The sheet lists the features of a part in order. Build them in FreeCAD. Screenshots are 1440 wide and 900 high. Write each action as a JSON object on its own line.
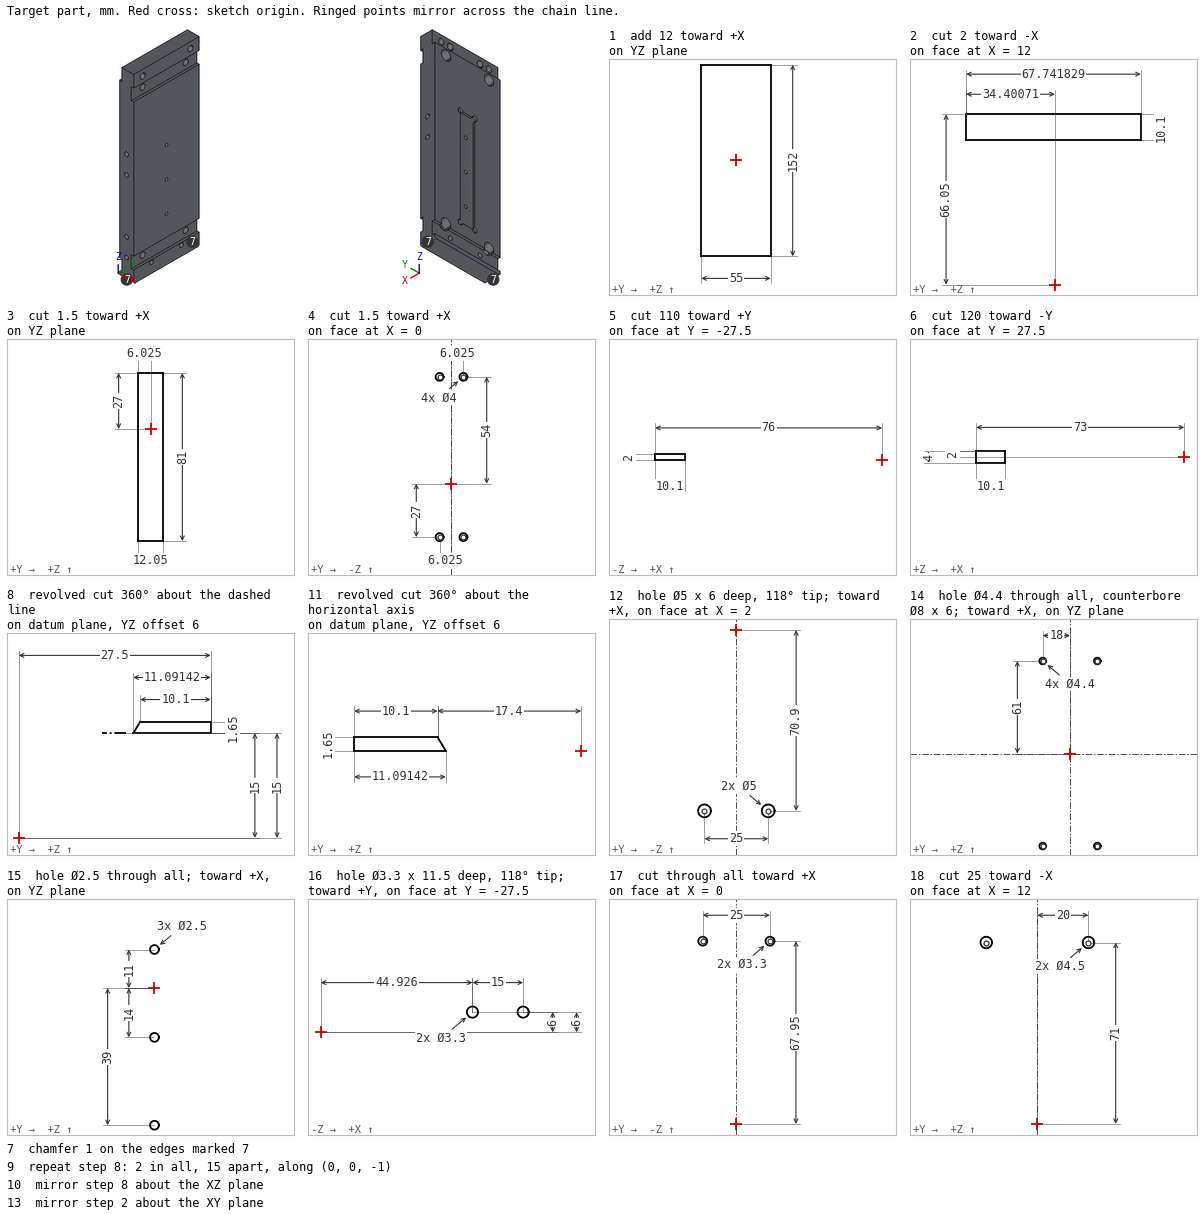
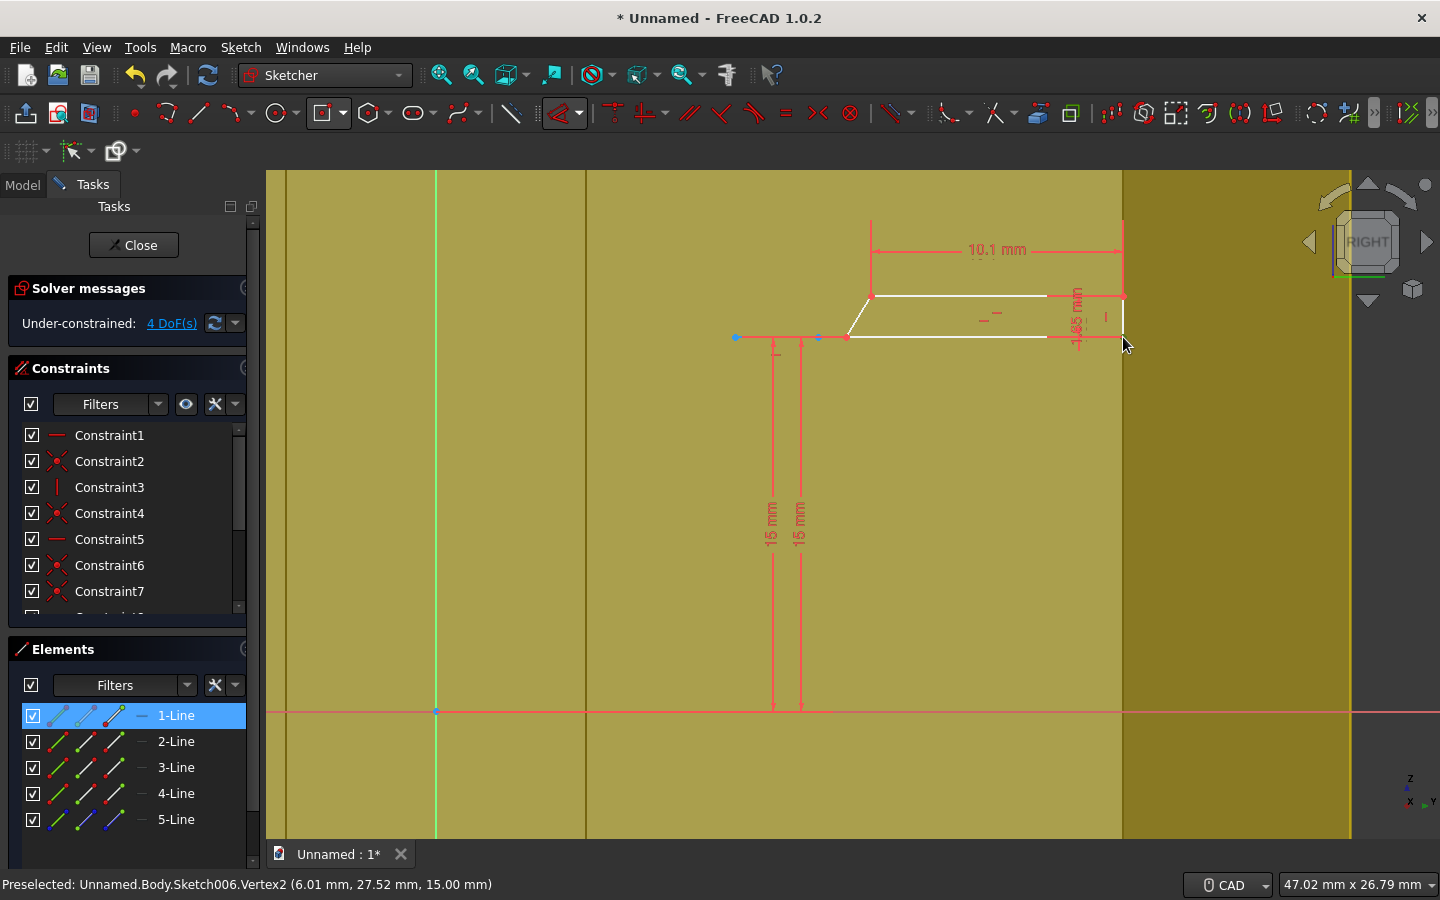
{"action": "left_click", "coordinate": [582, 114]}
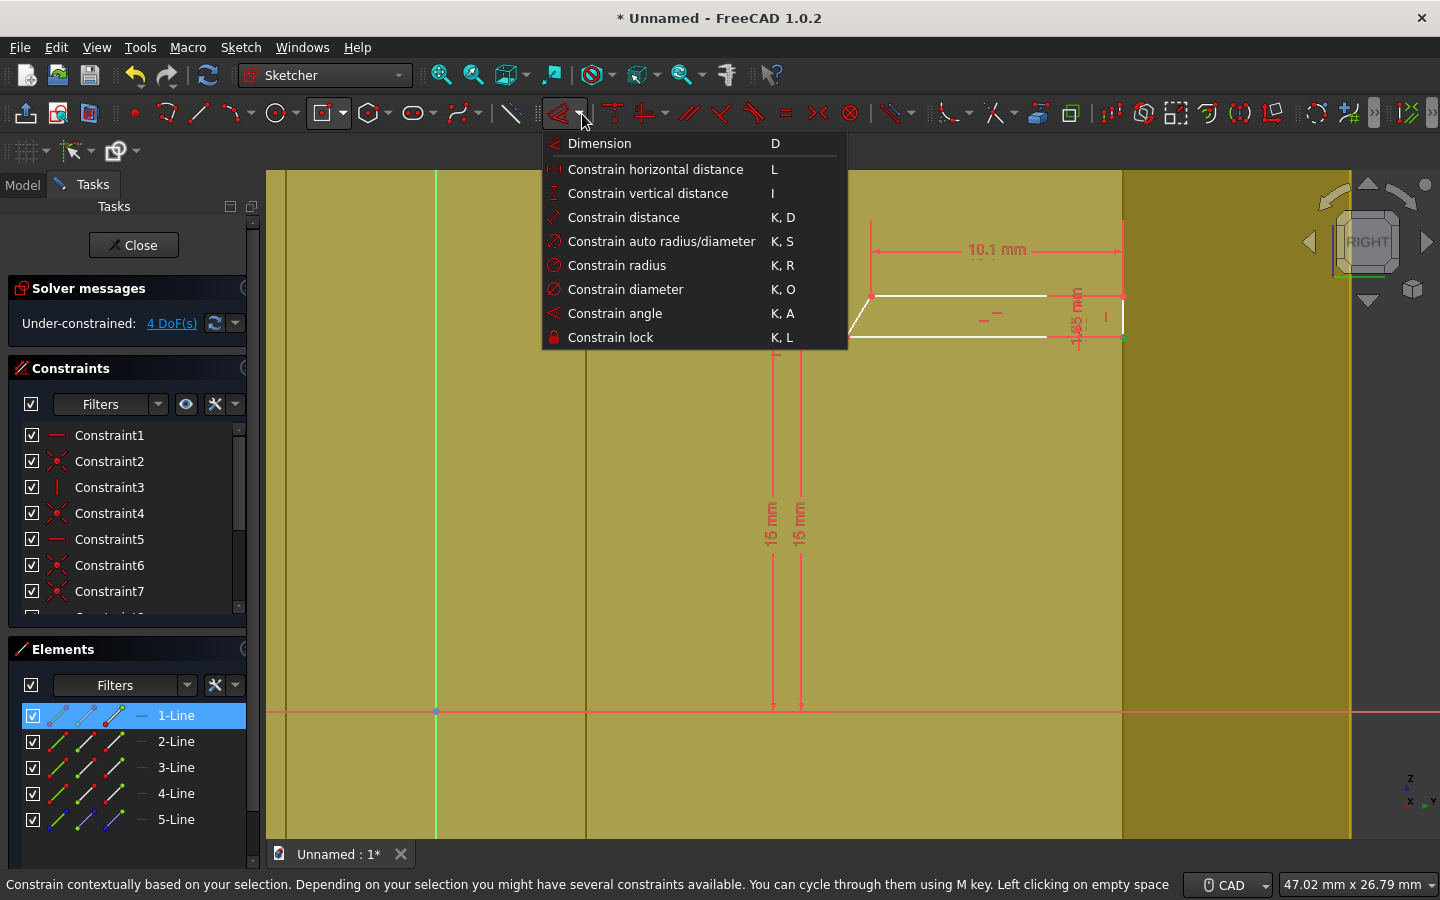
{"action": "left_click", "coordinate": [695, 169]}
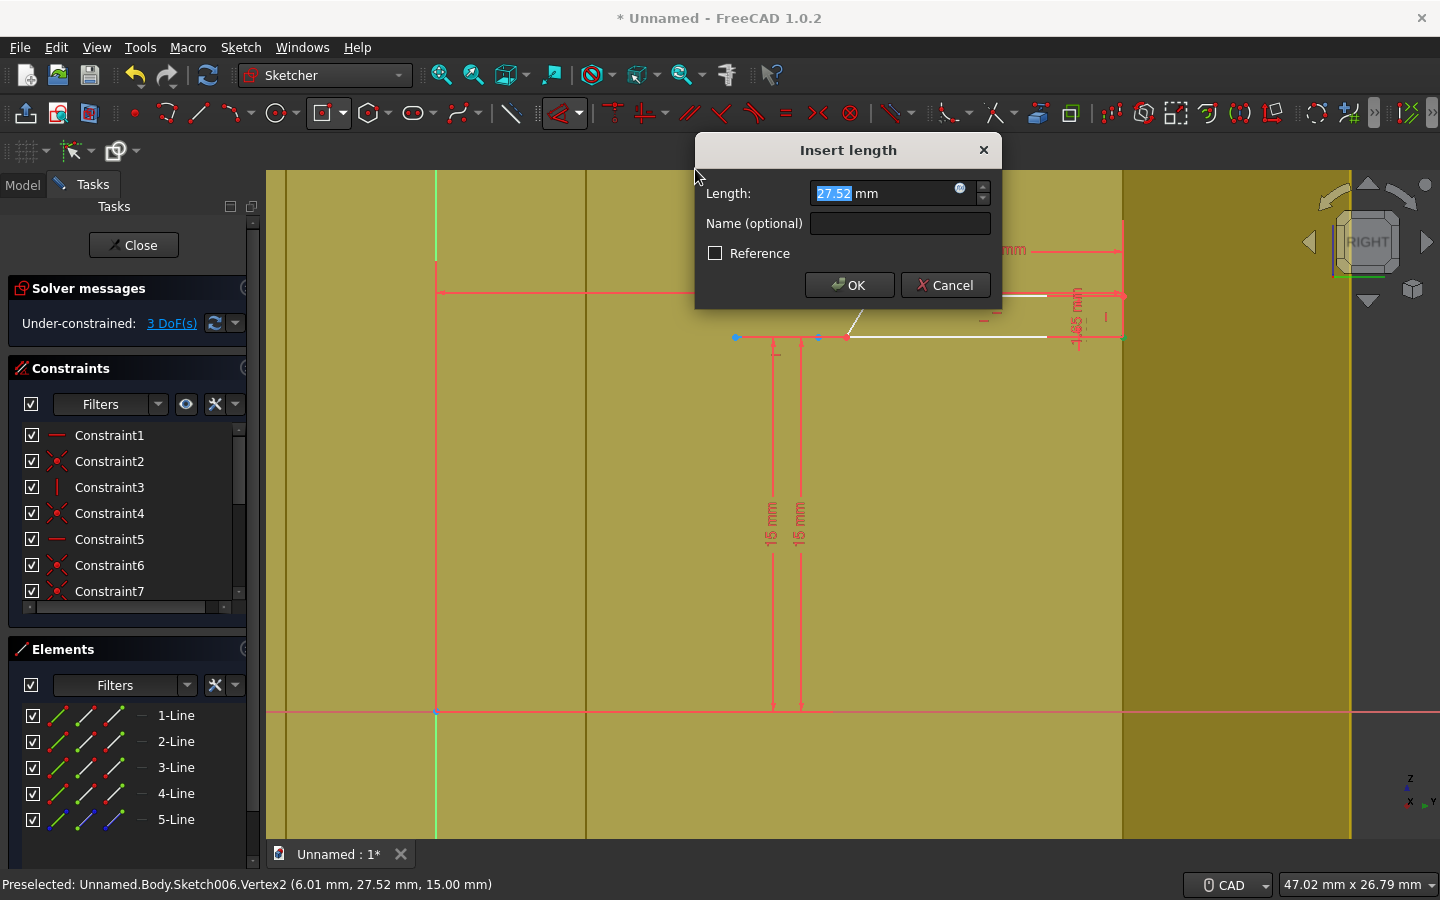
{"action": "type", "text": "27.5"}
{"action": "key", "text": "Return"}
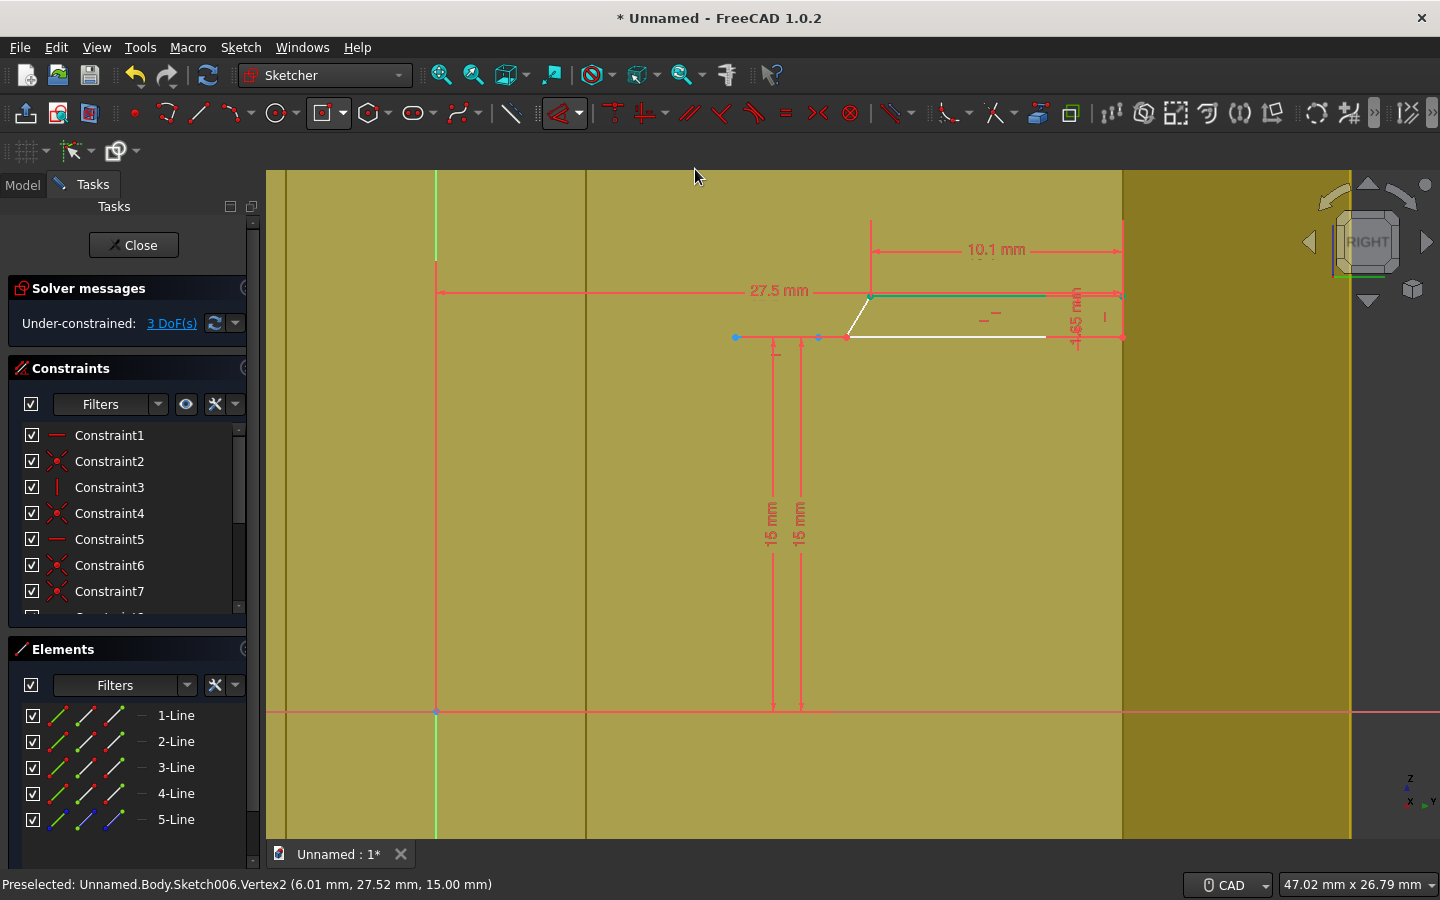
{"action": "left_click", "coordinate": [929, 337]}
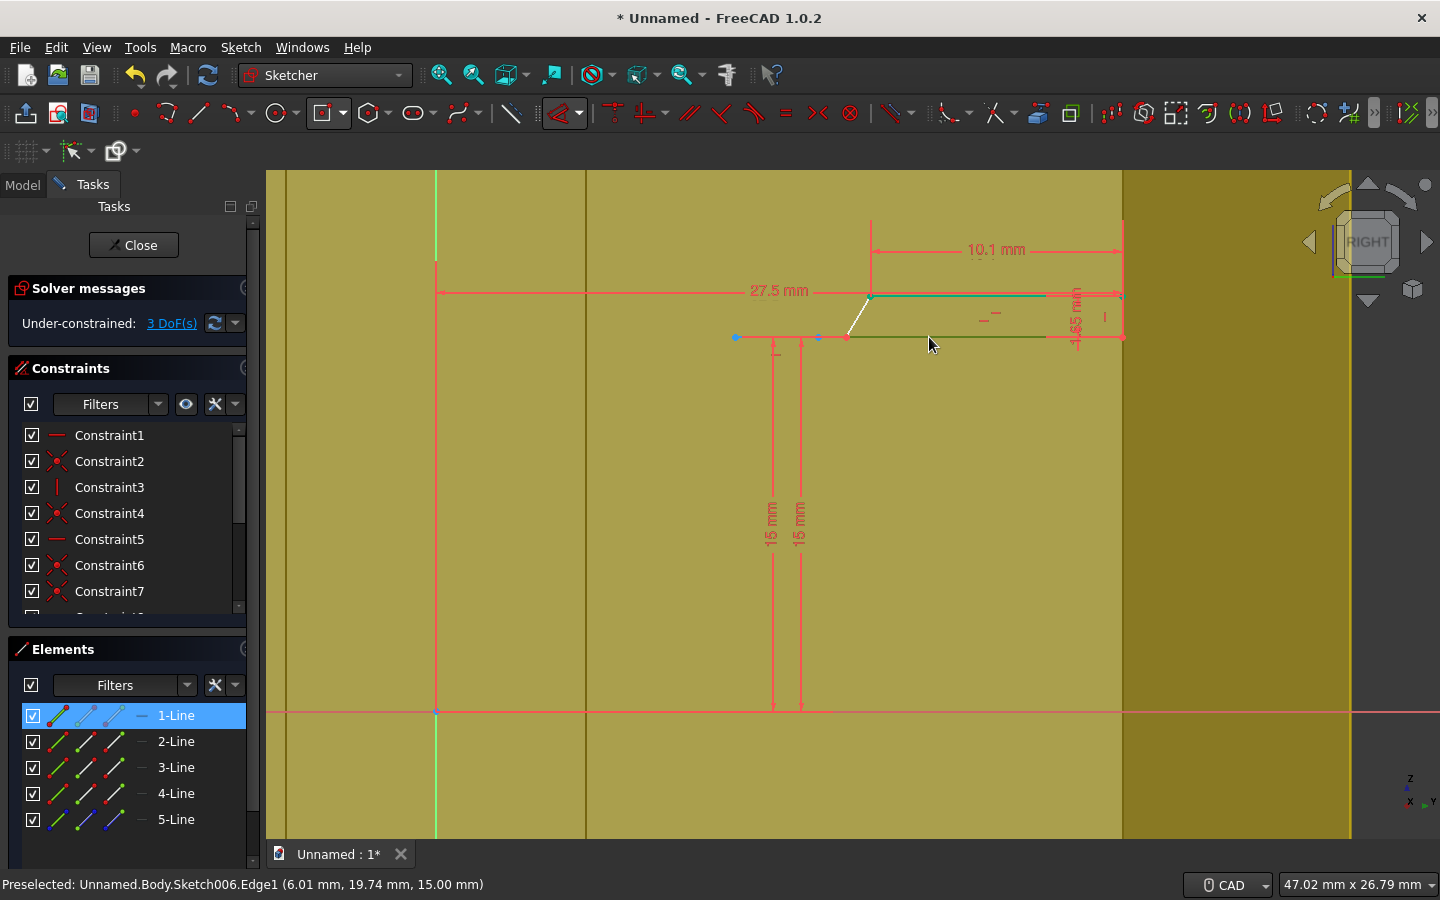
{"action": "left_click", "coordinate": [582, 114]}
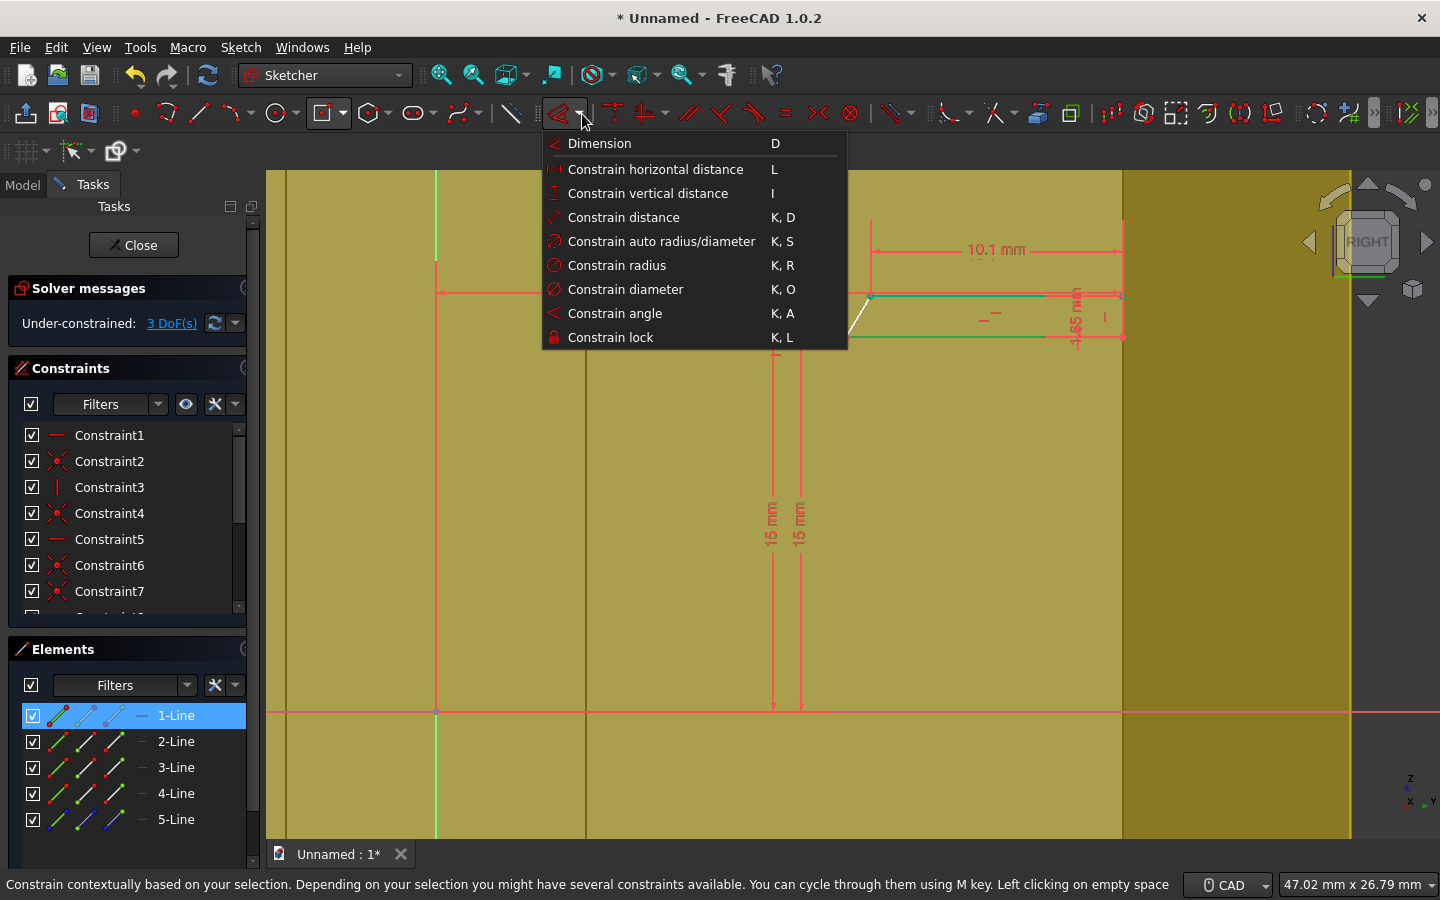
{"action": "left_click", "coordinate": [695, 169]}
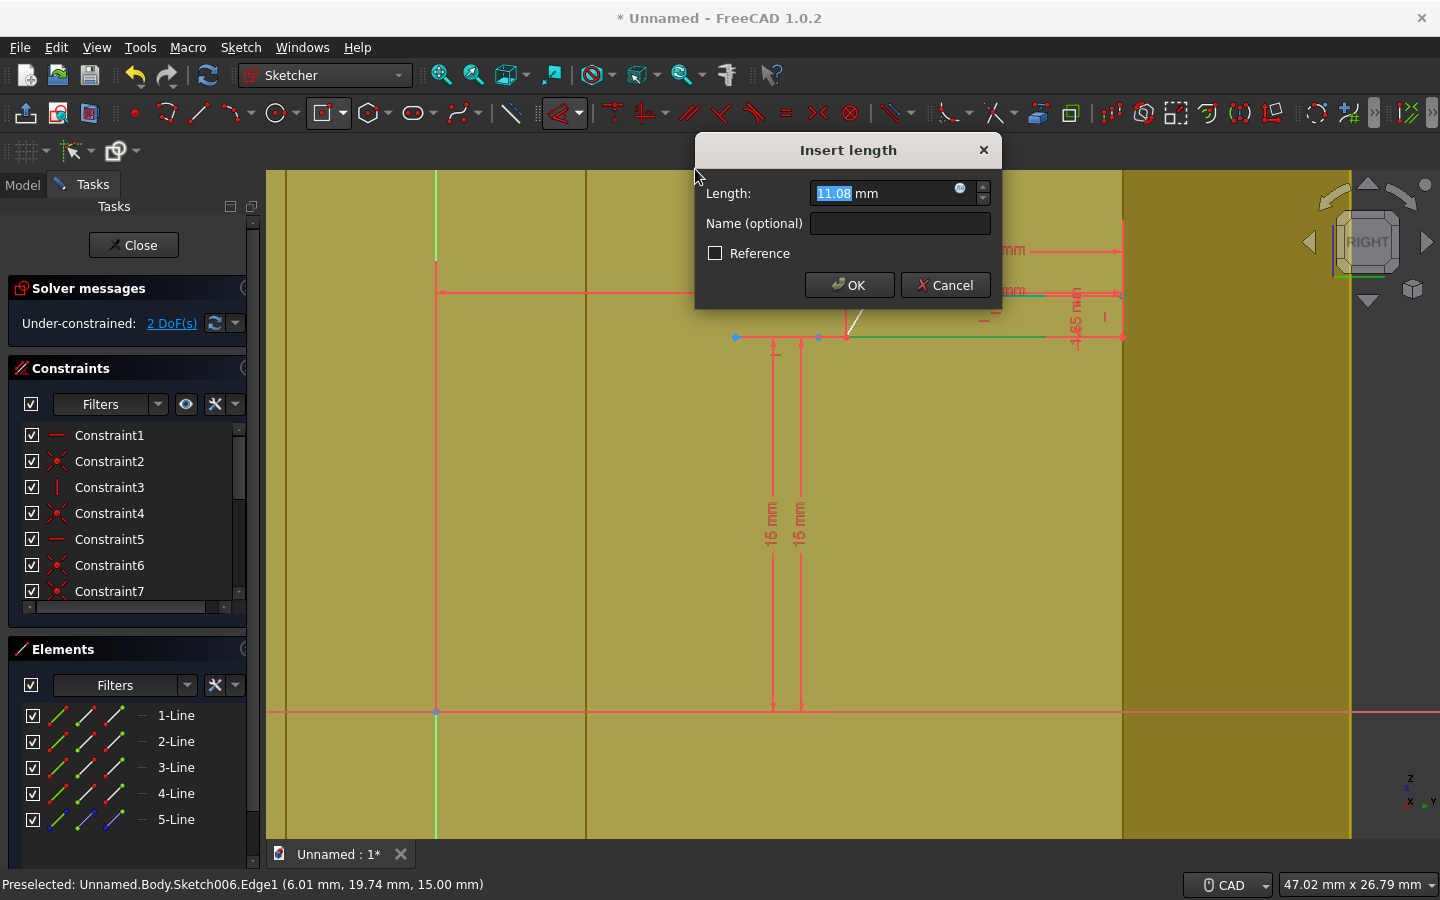
{"action": "type", "text": "11.09142"}
{"action": "key", "text": "Return"}